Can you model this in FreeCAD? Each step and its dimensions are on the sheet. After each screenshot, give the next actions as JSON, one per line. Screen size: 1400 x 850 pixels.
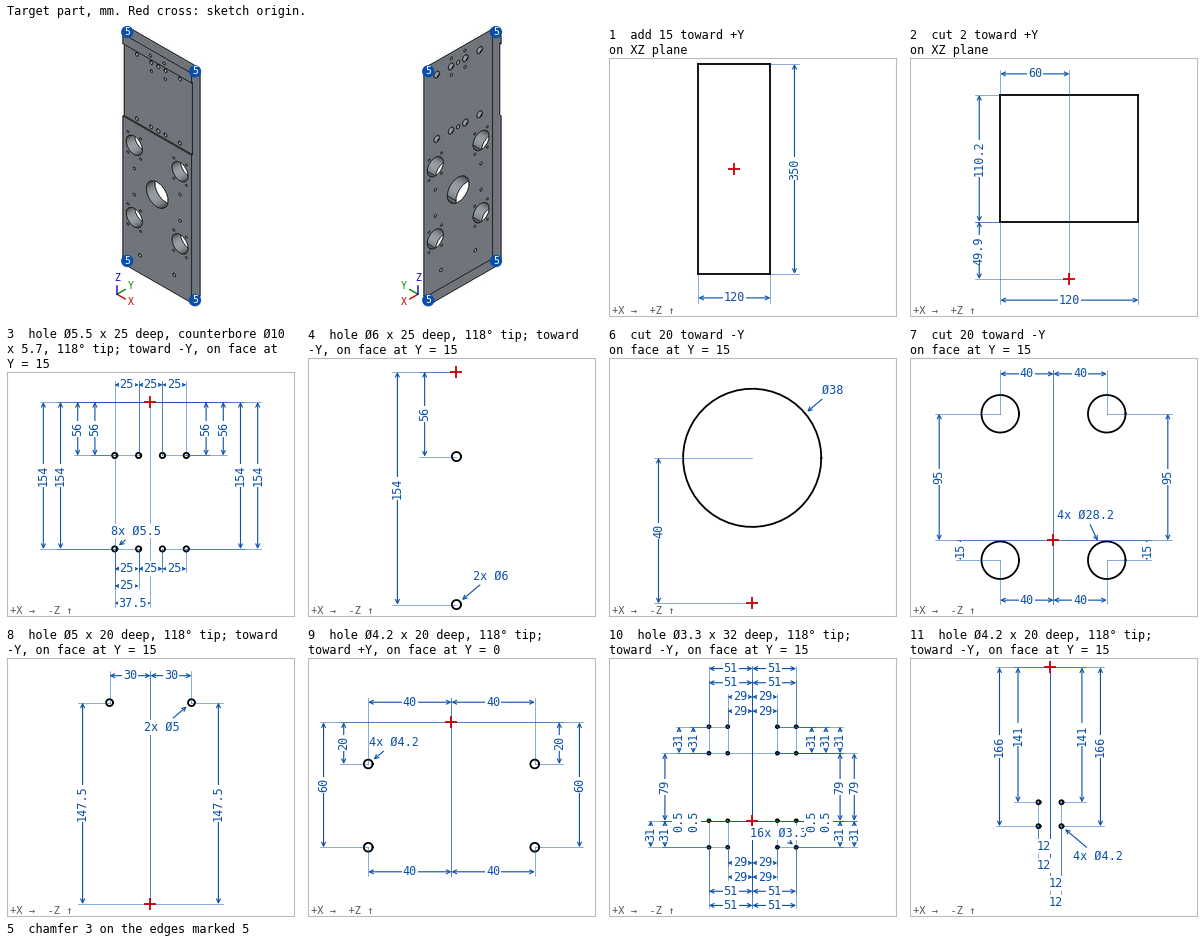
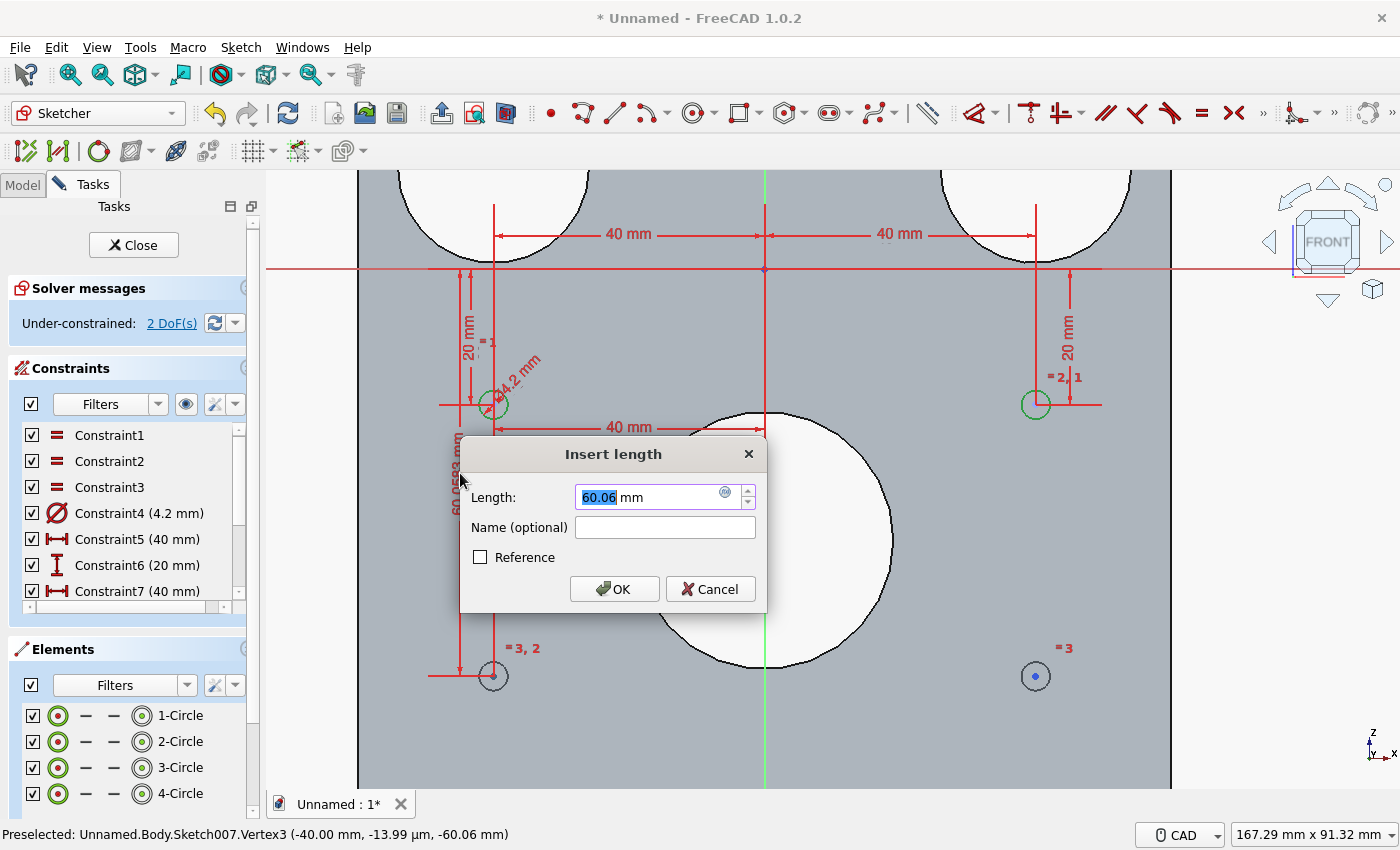
{"action": "type", "text": "60"}
{"action": "key", "text": "Return"}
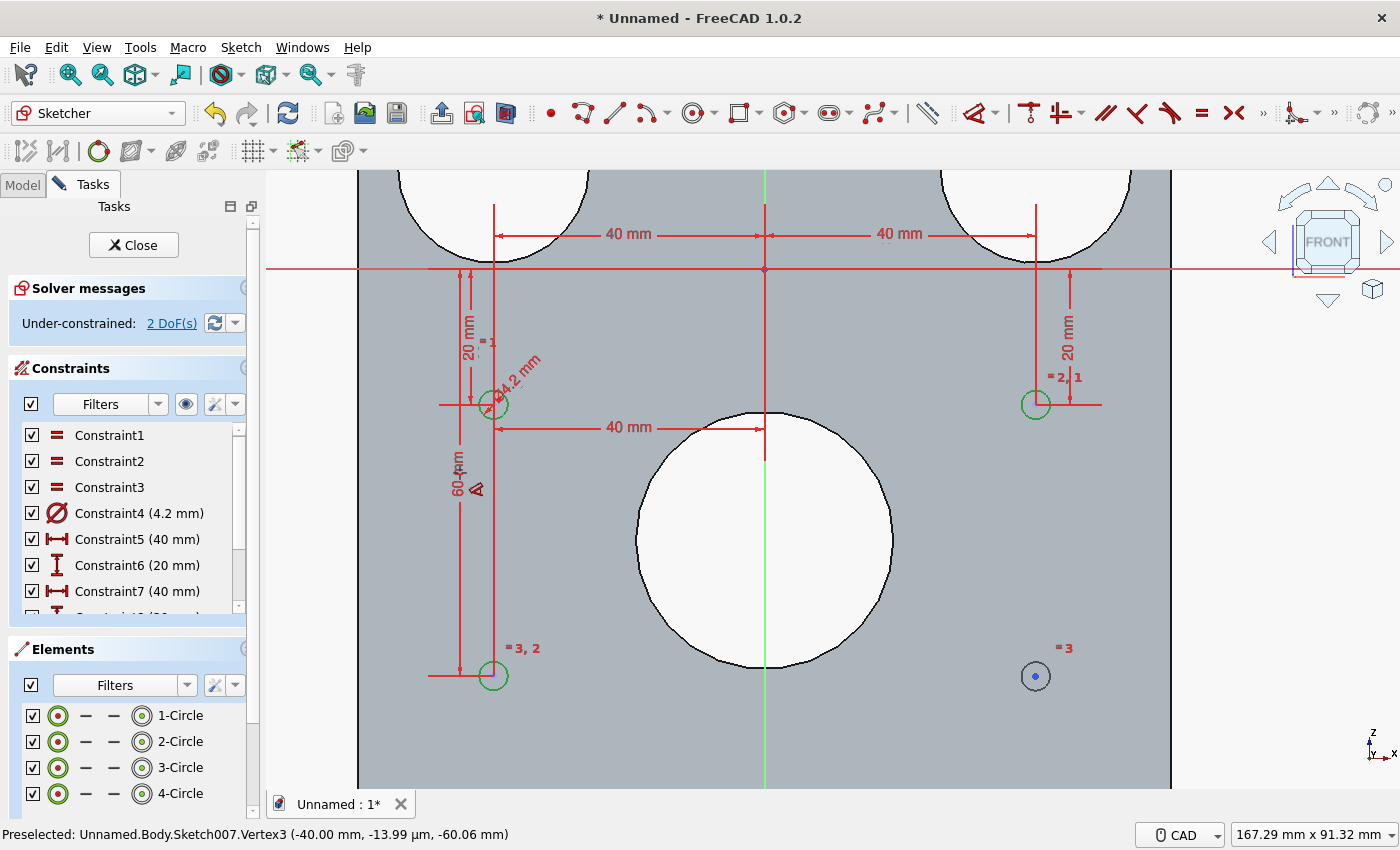
{"action": "left_click", "coordinate": [1036, 676]}
{"action": "left_click", "coordinate": [805, 235]}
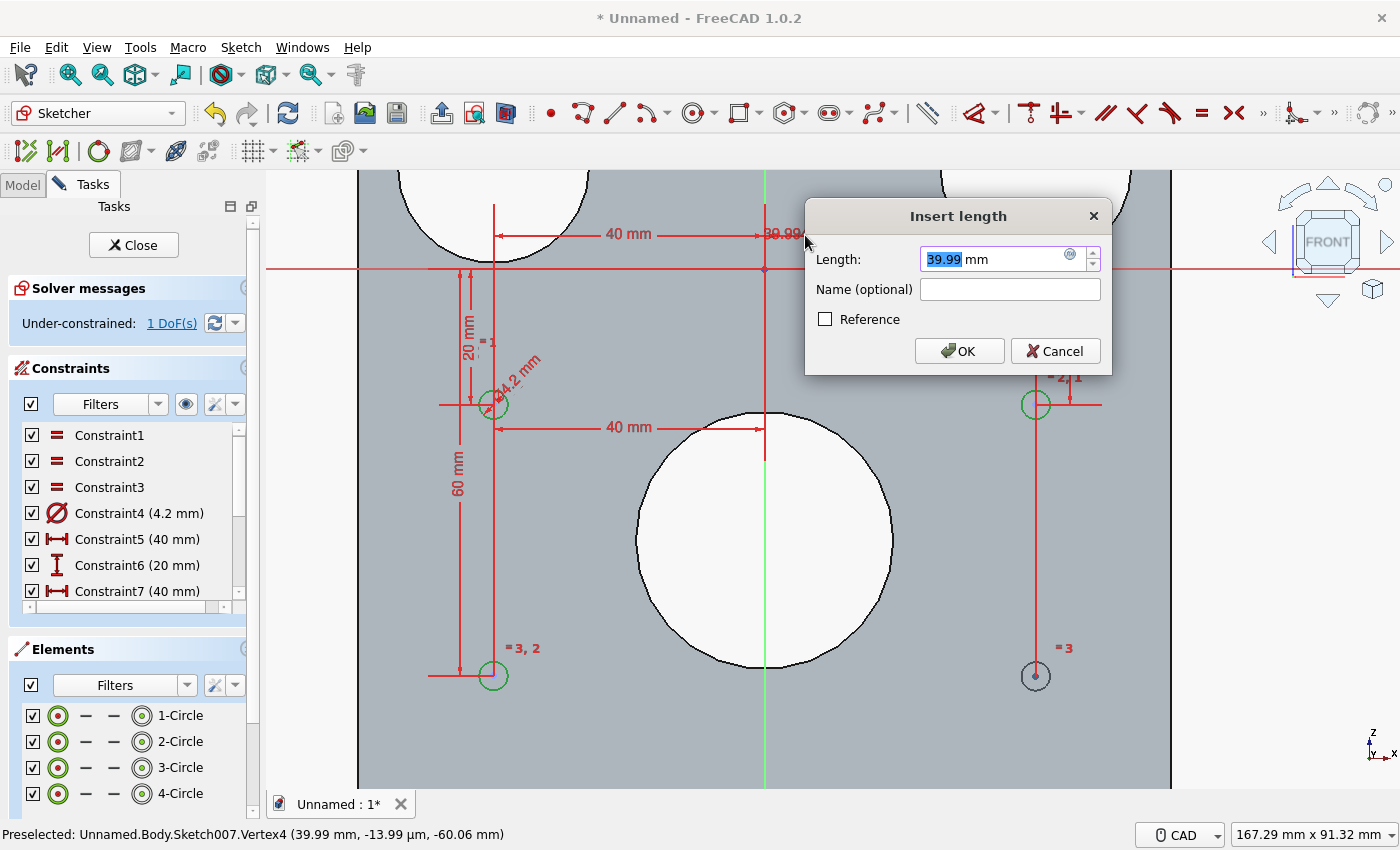
{"action": "type", "text": "40"}
{"action": "key", "text": "Return"}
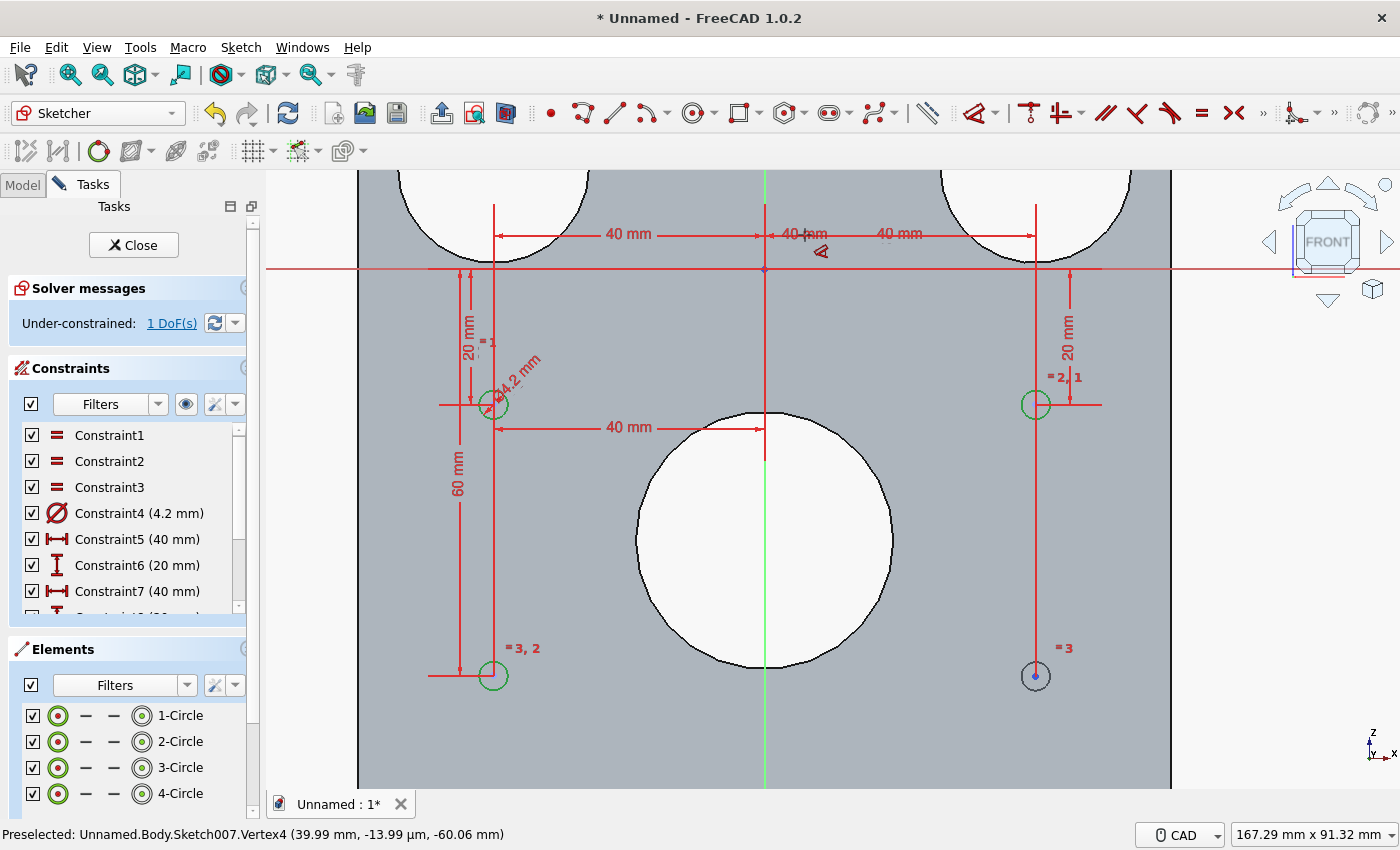
{"action": "left_click", "coordinate": [1036, 676]}
{"action": "left_click", "coordinate": [1070, 473]}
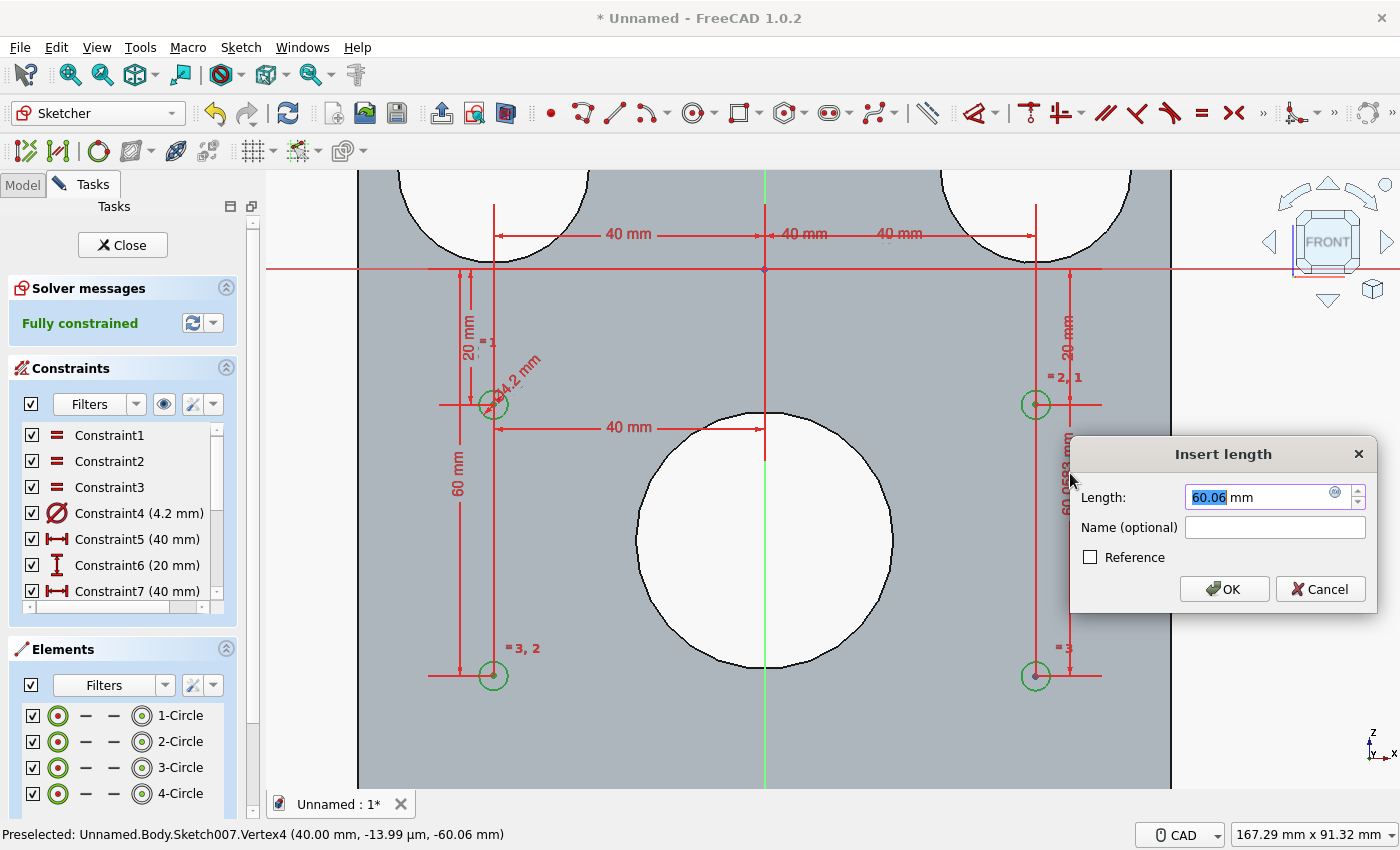
{"action": "type", "text": "60"}
{"action": "key", "text": "Return"}
{"action": "key", "text": "Escape"}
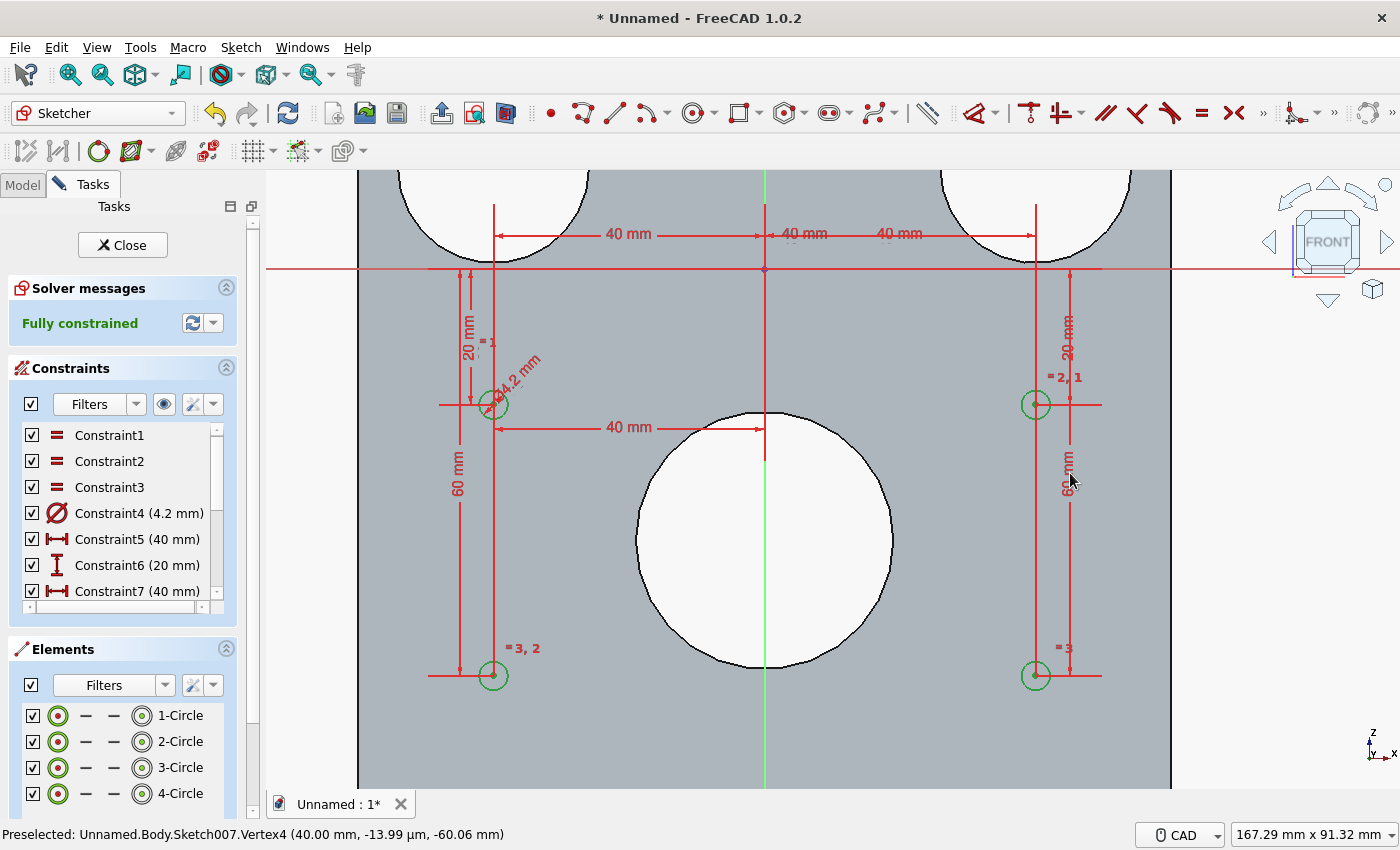
{"action": "left_click", "coordinate": [123, 245]}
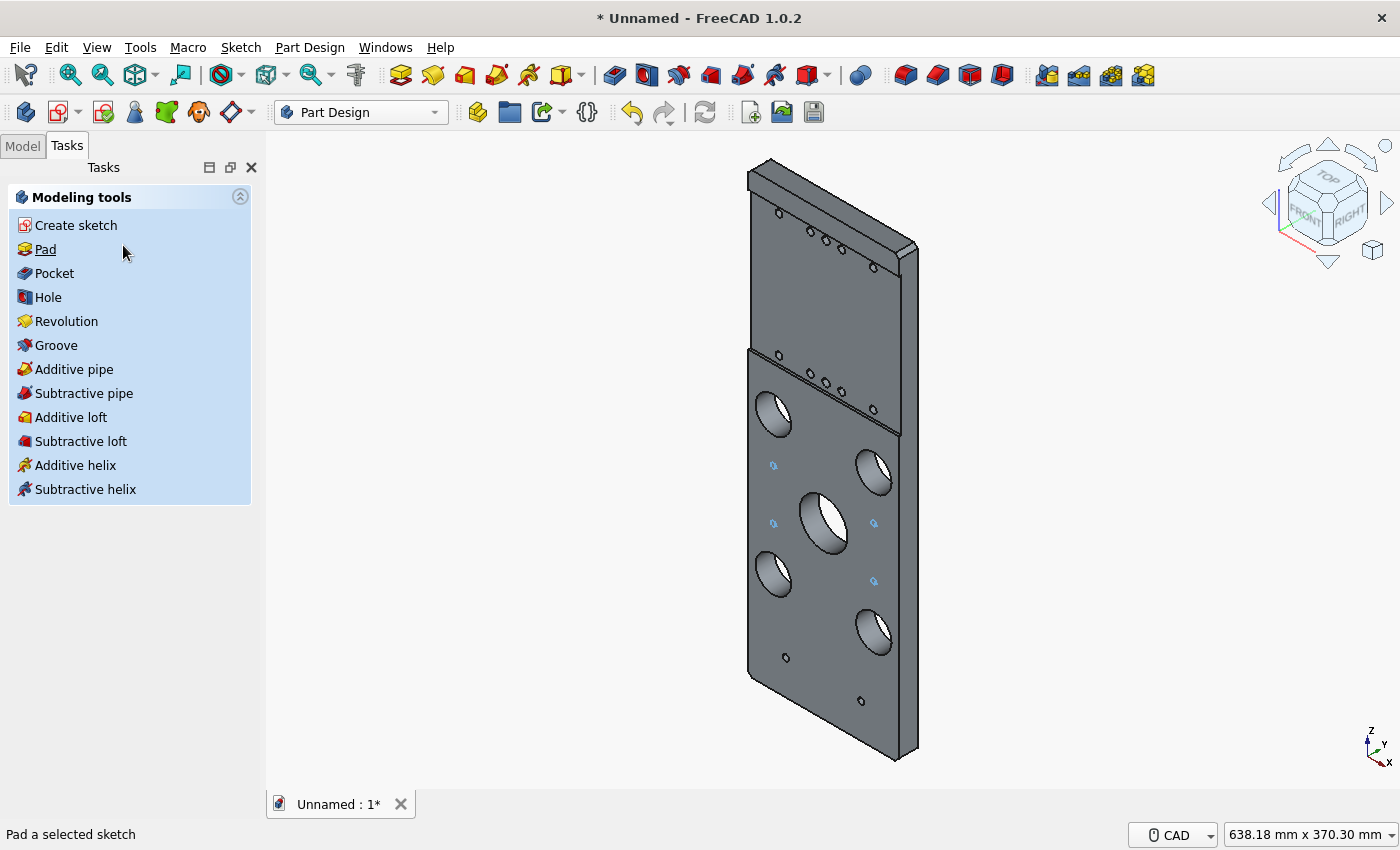
{"action": "left_click", "coordinate": [648, 76]}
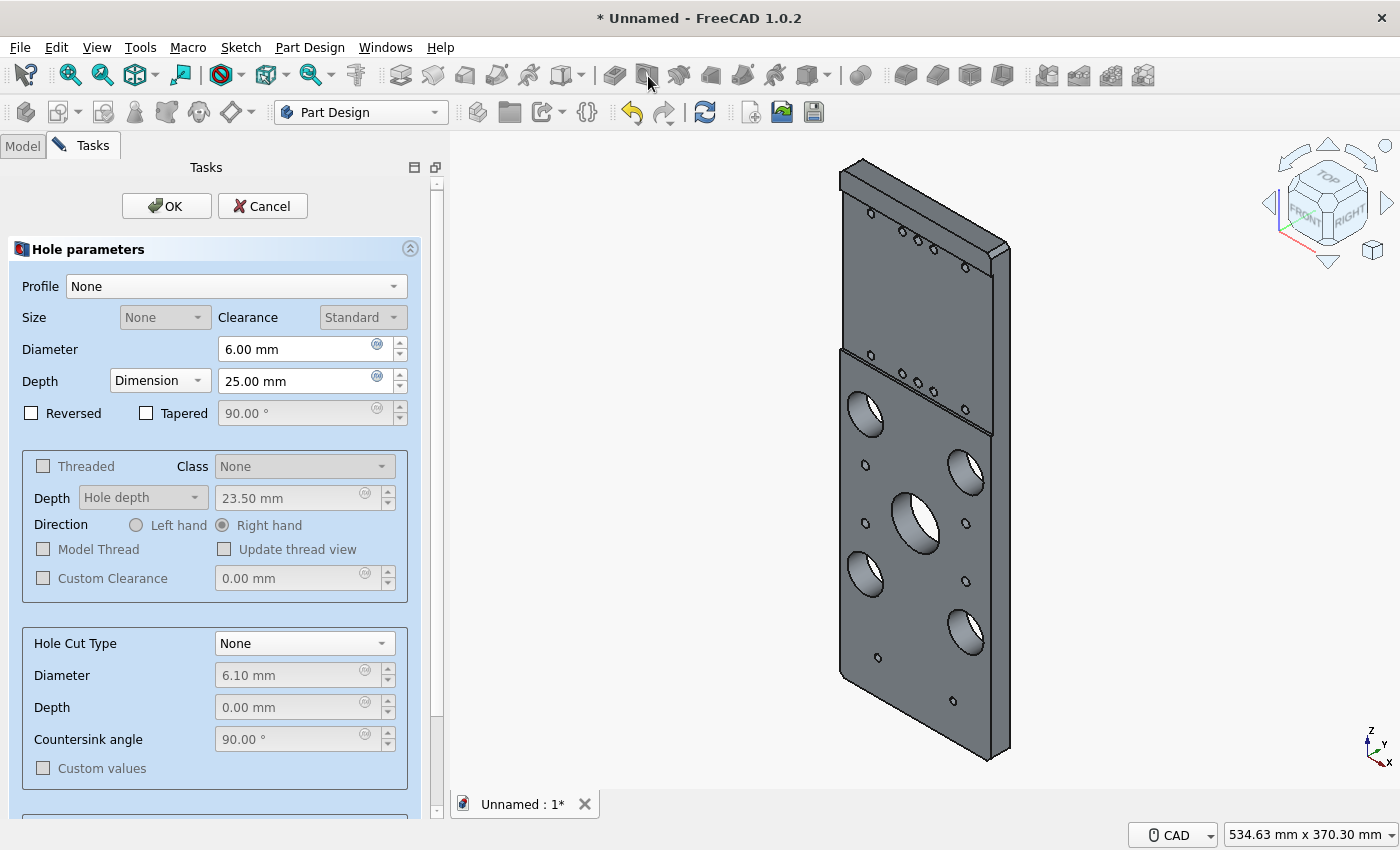
{"action": "triple_click", "coordinate": [305, 349]}